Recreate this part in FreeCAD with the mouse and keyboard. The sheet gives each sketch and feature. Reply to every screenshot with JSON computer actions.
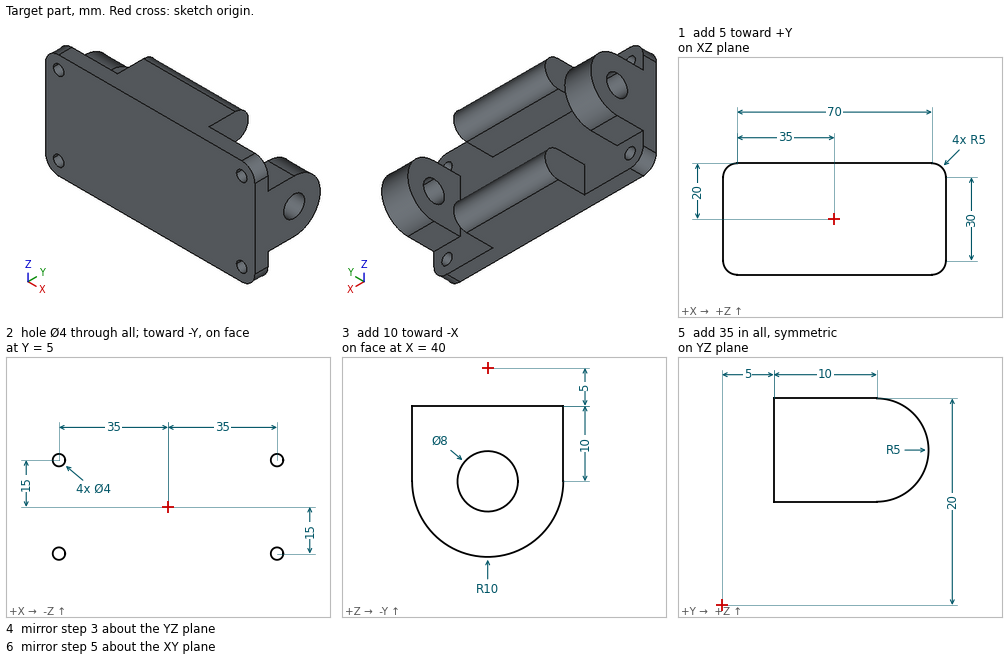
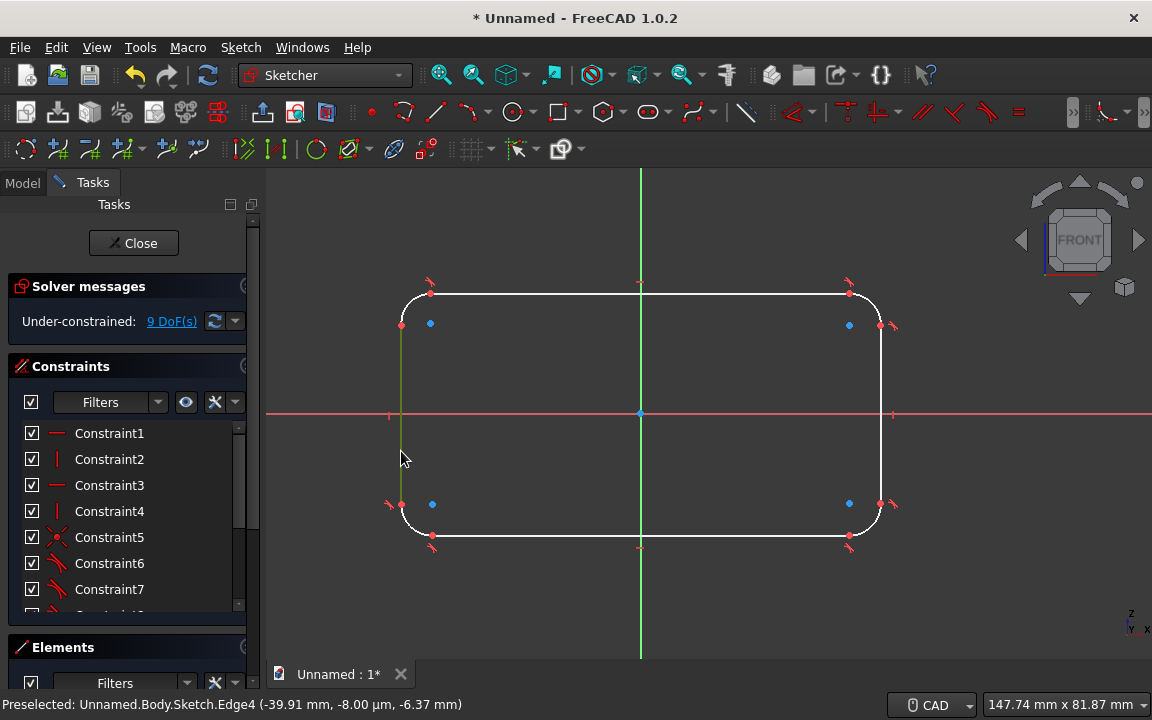
{"action": "left_click", "coordinate": [417, 297]}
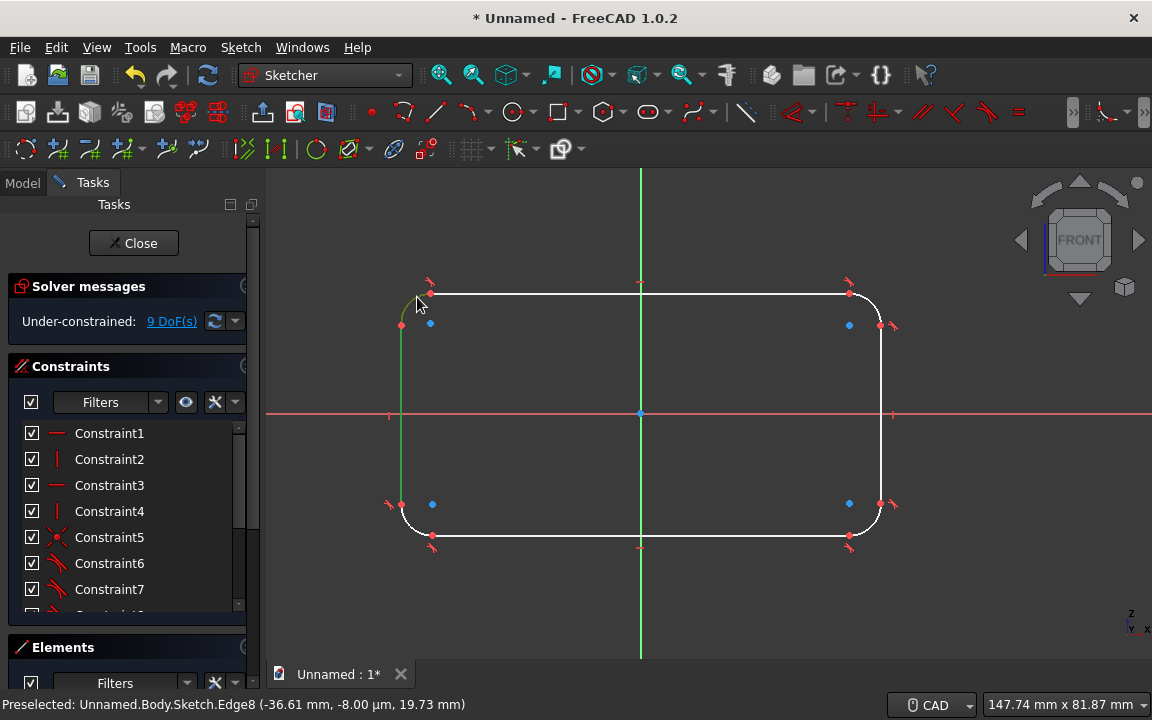
{"action": "key", "text": "t"}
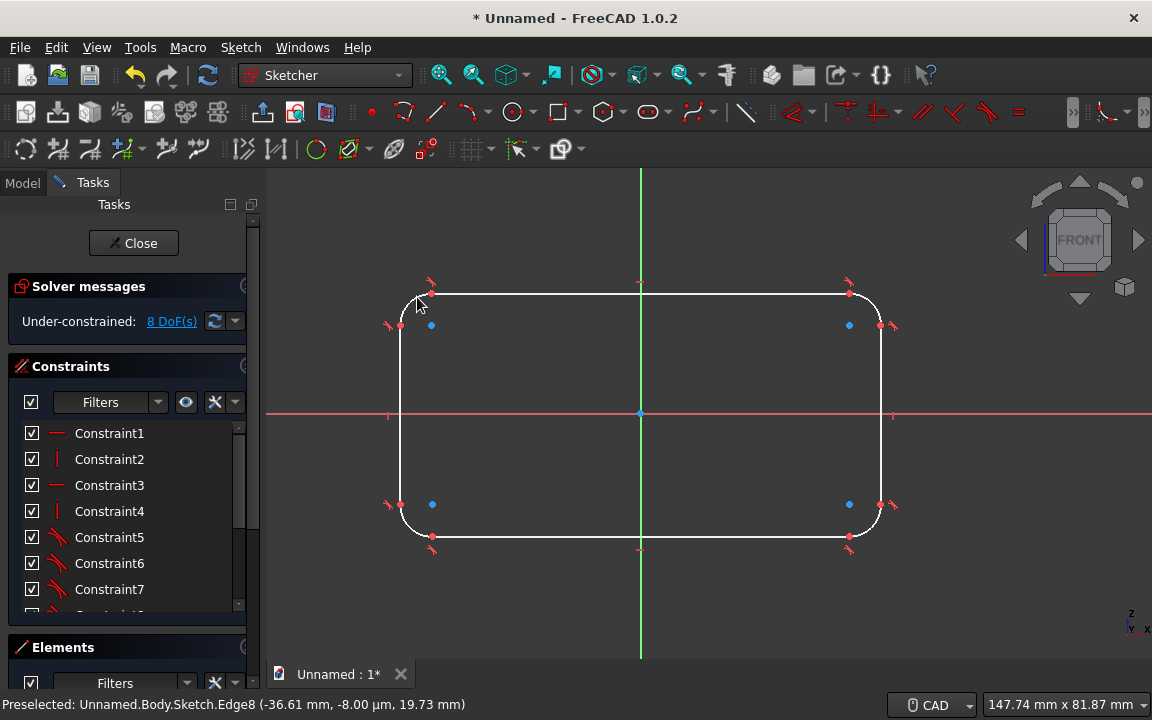
{"action": "left_click", "coordinate": [878, 311]}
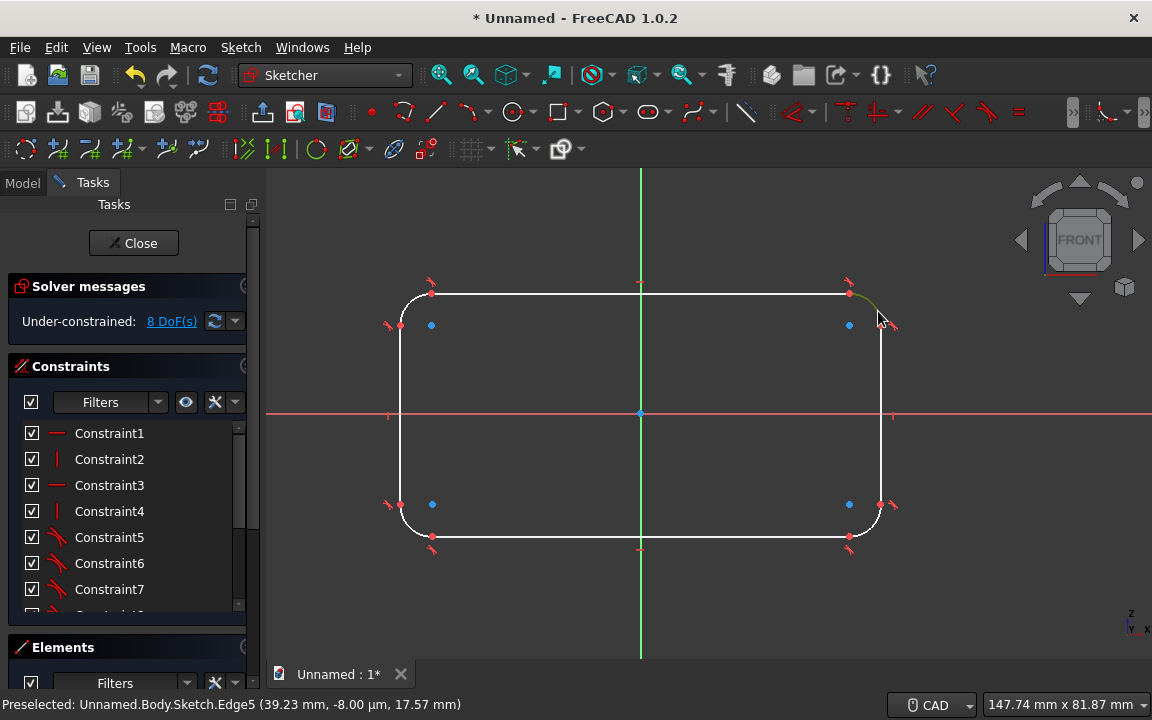
{"action": "left_click", "coordinate": [864, 533]}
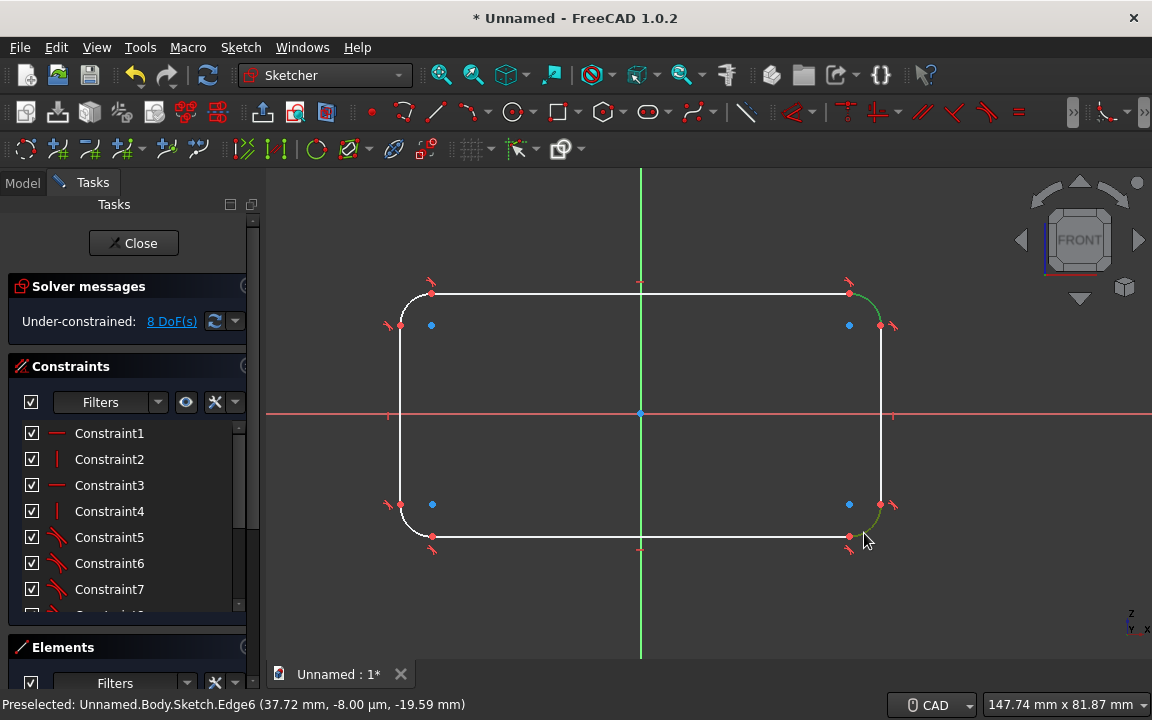
{"action": "left_click", "coordinate": [404, 519]}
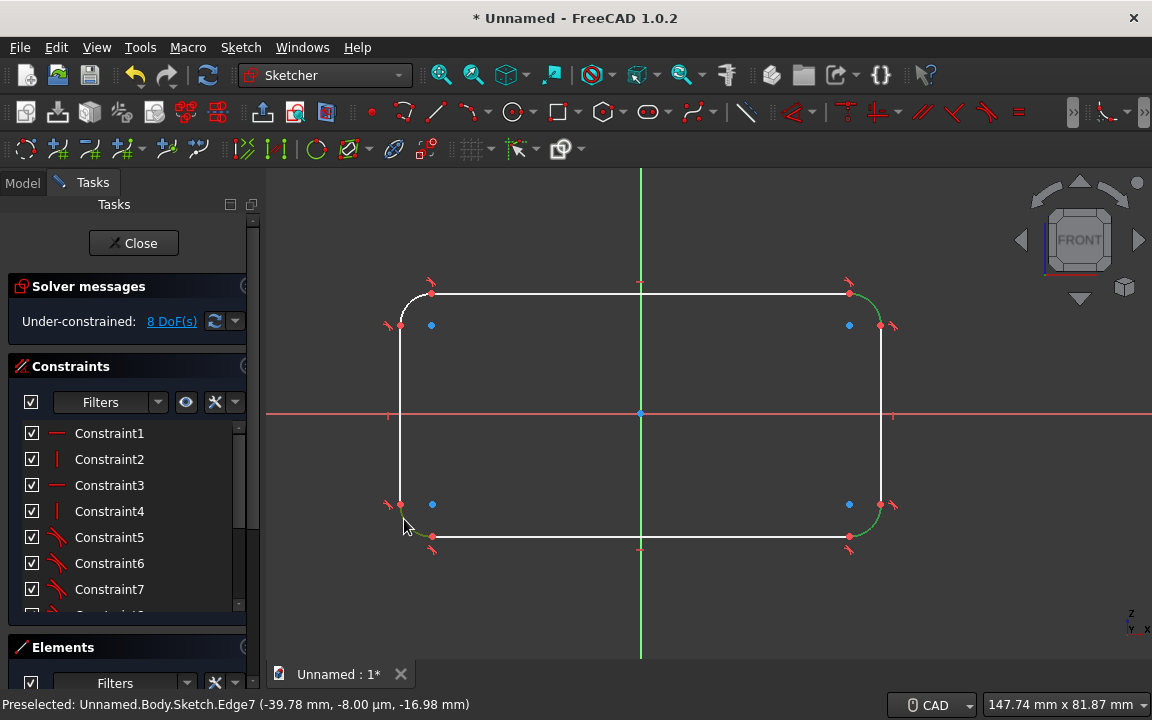
{"action": "left_click", "coordinate": [417, 297]}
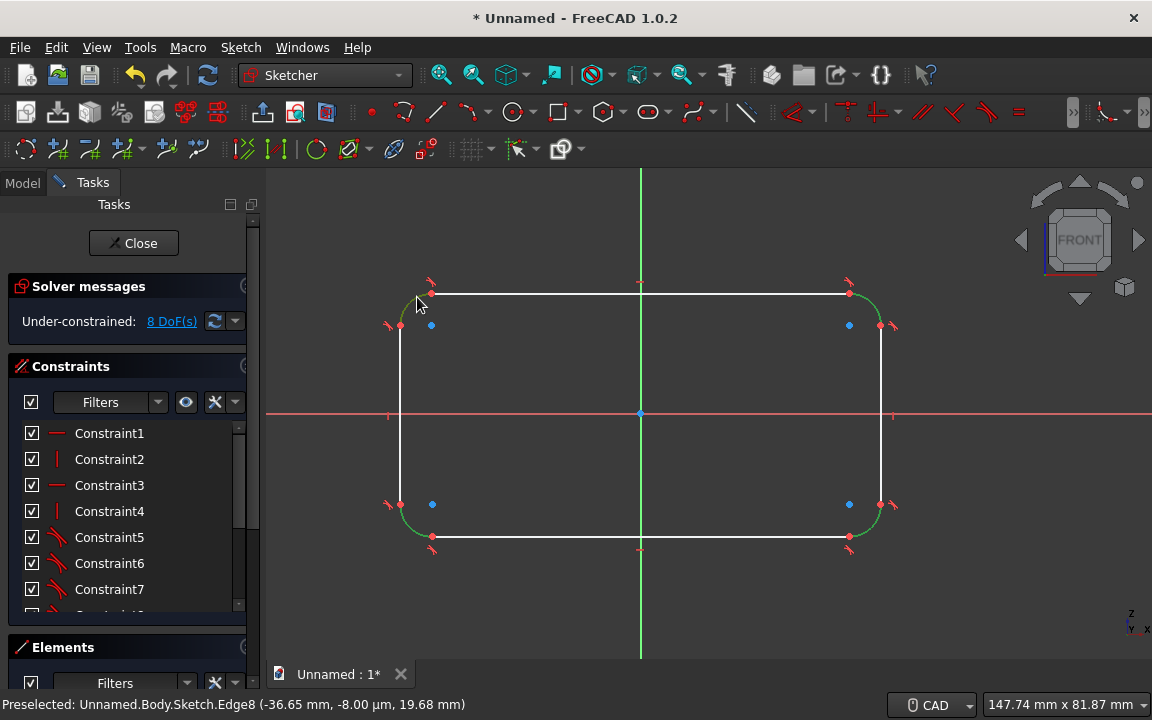
{"action": "key", "text": "e"}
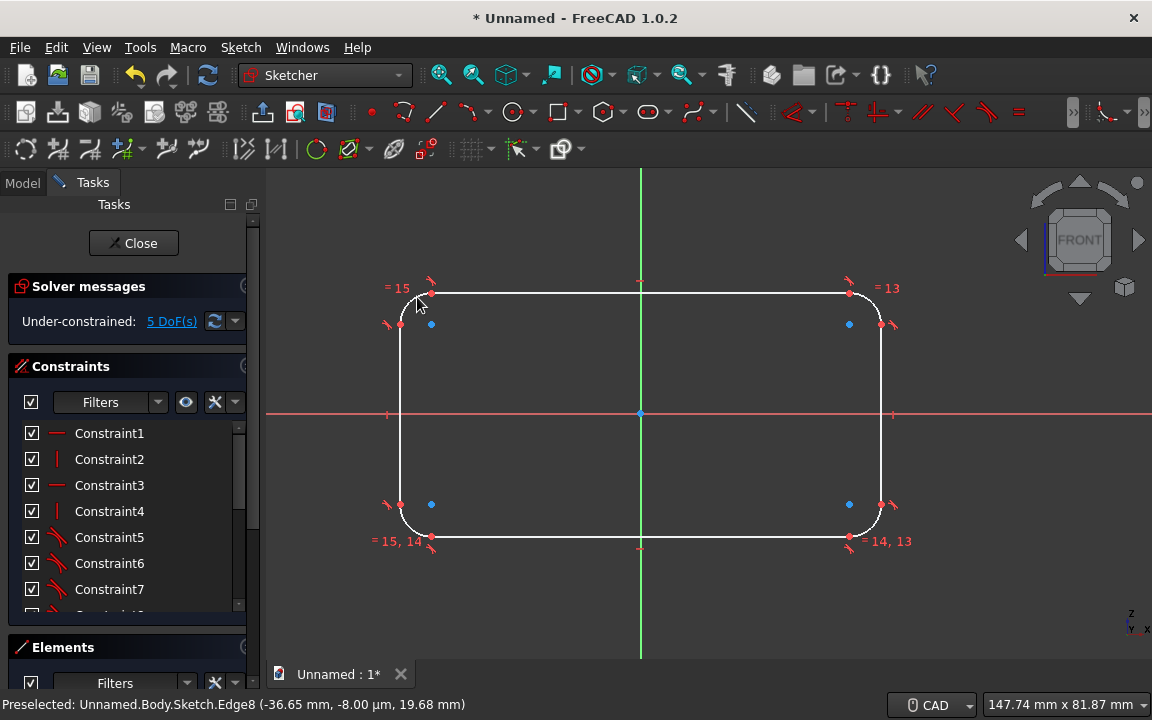
{"action": "scroll", "coordinate": [878, 310], "scroll_direction": "up", "scroll_amount": 2}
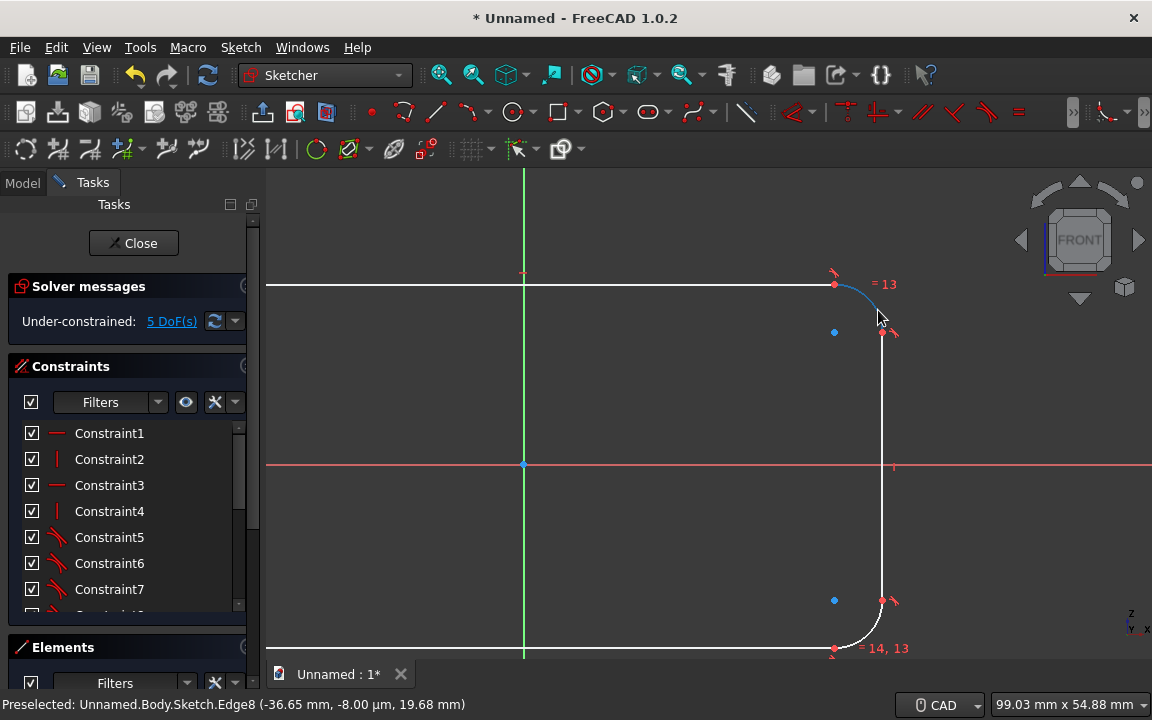
{"action": "left_click", "coordinate": [877, 311]}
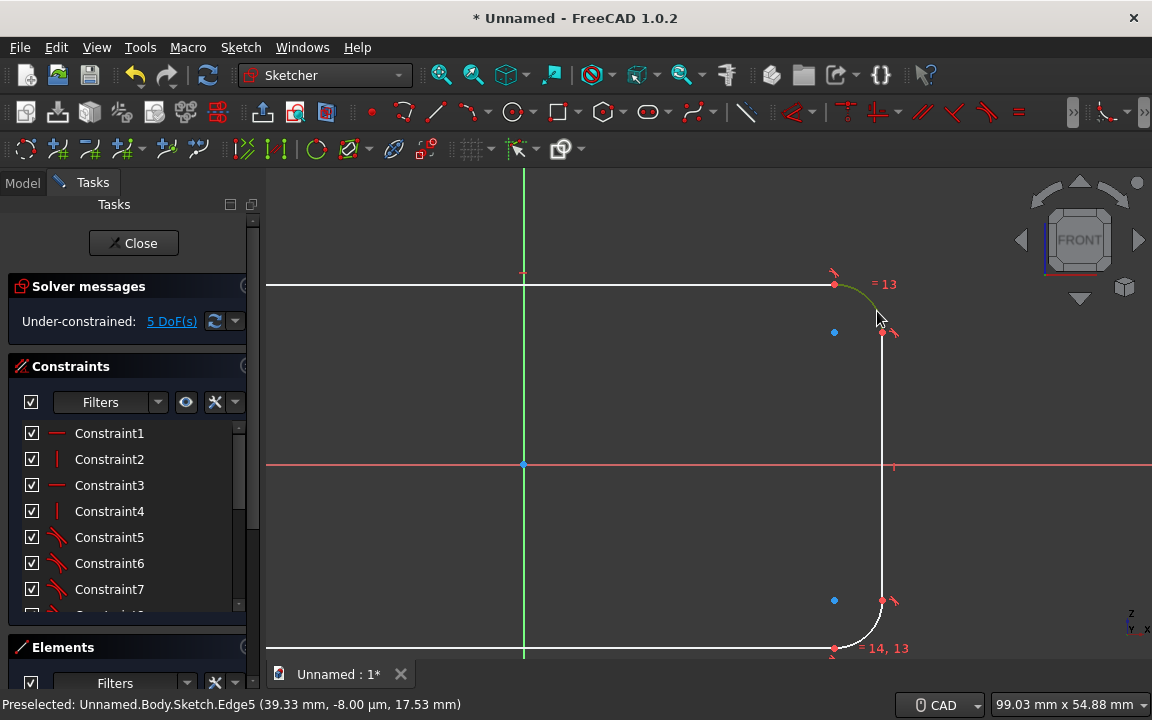
{"action": "key", "text": "k r"}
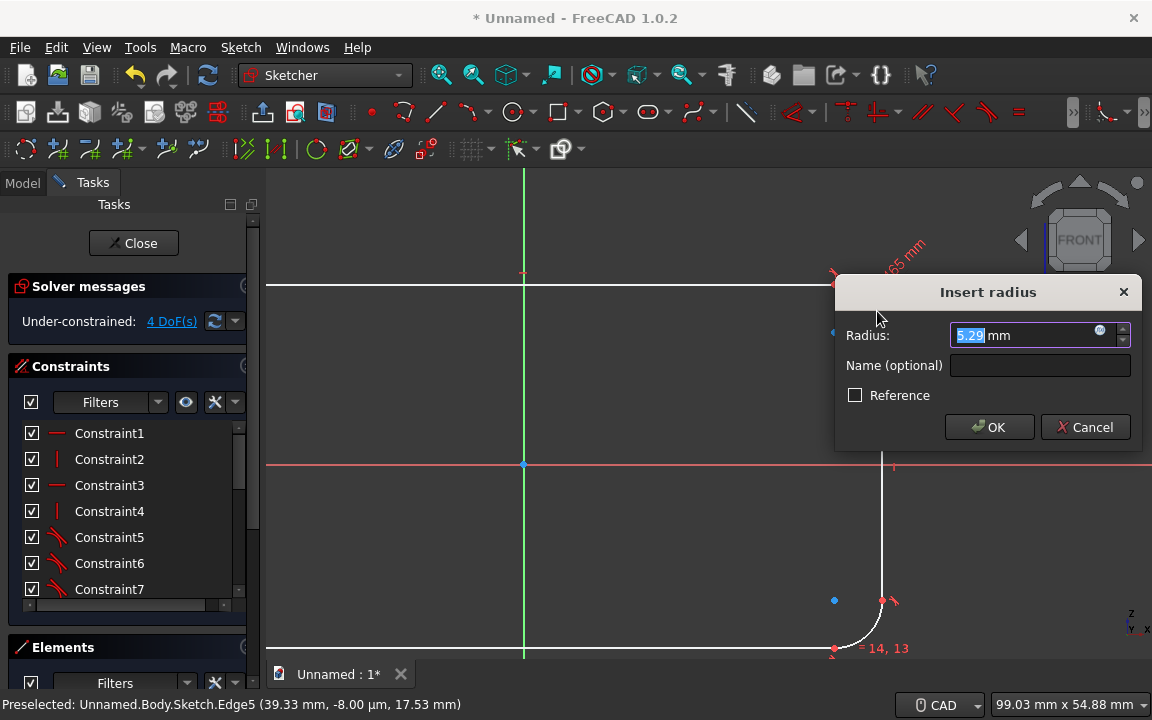
{"action": "type", "text": "5"}
{"action": "key", "text": "Return"}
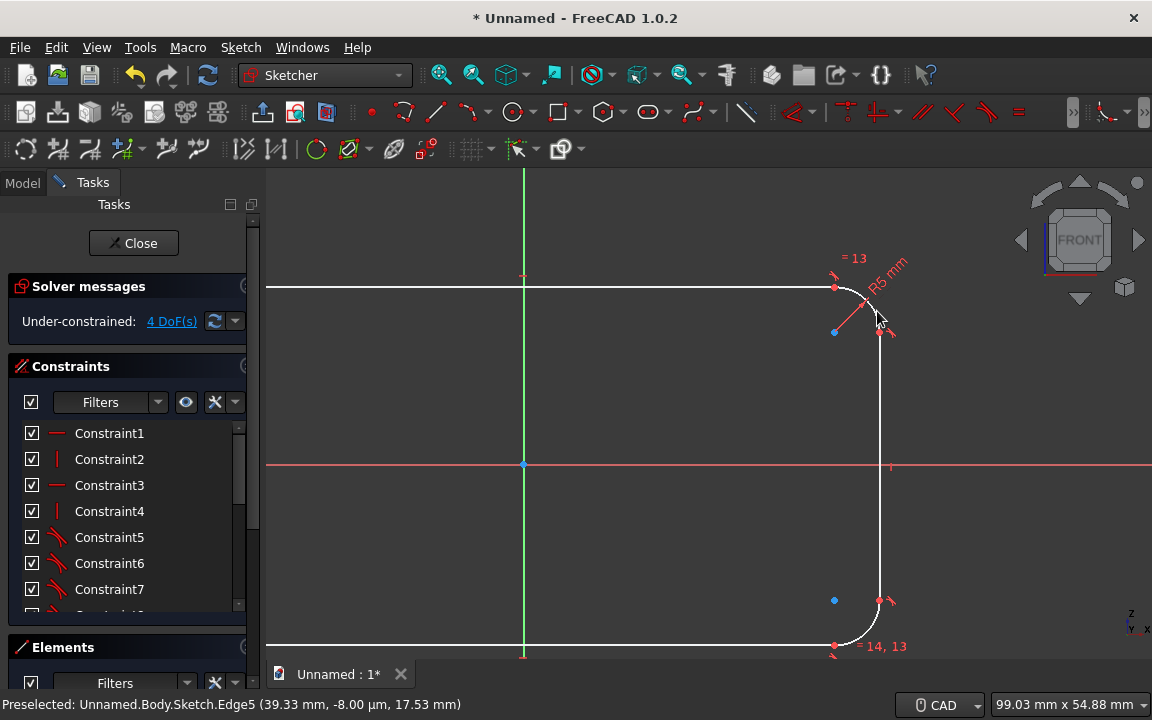
{"action": "left_click", "coordinate": [399, 287]}